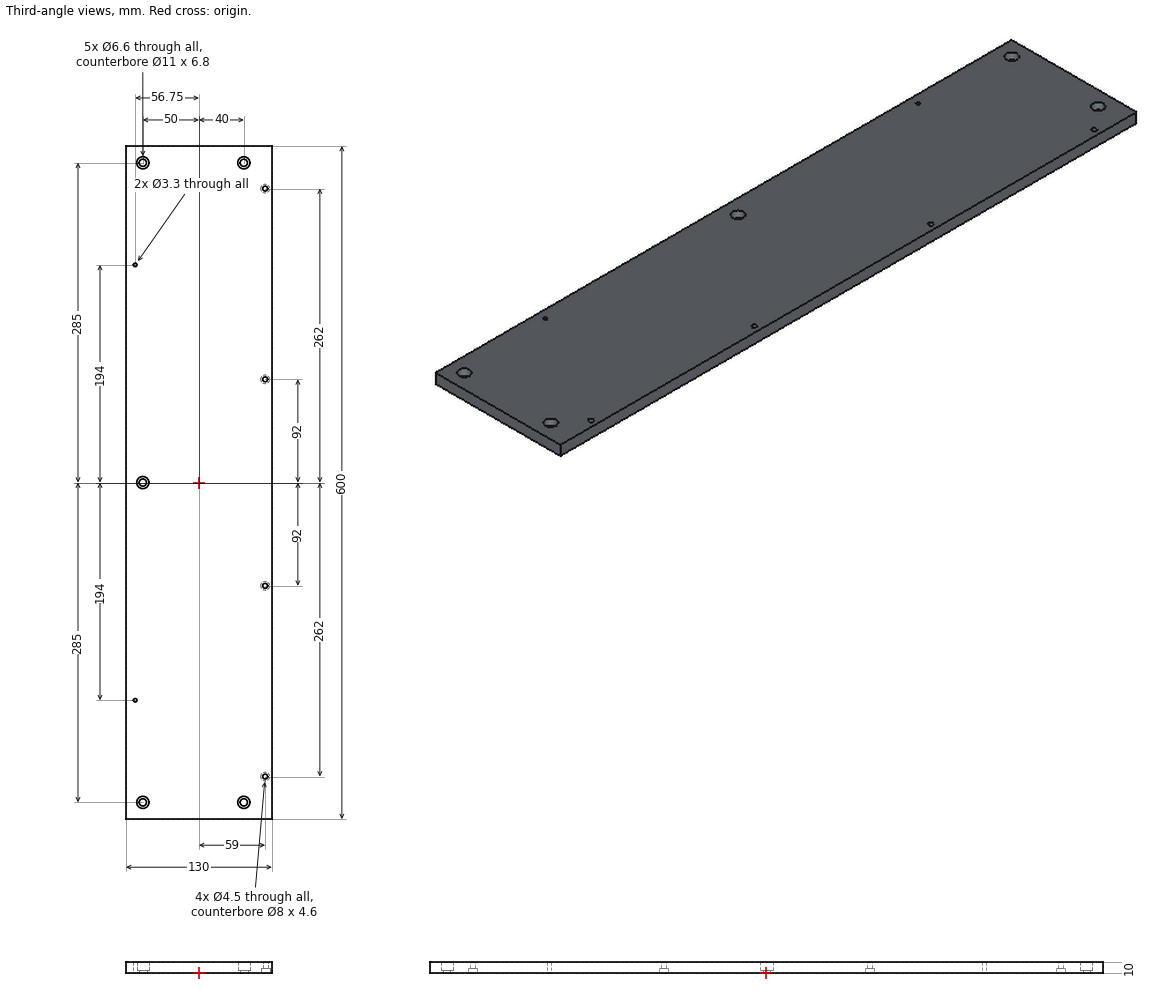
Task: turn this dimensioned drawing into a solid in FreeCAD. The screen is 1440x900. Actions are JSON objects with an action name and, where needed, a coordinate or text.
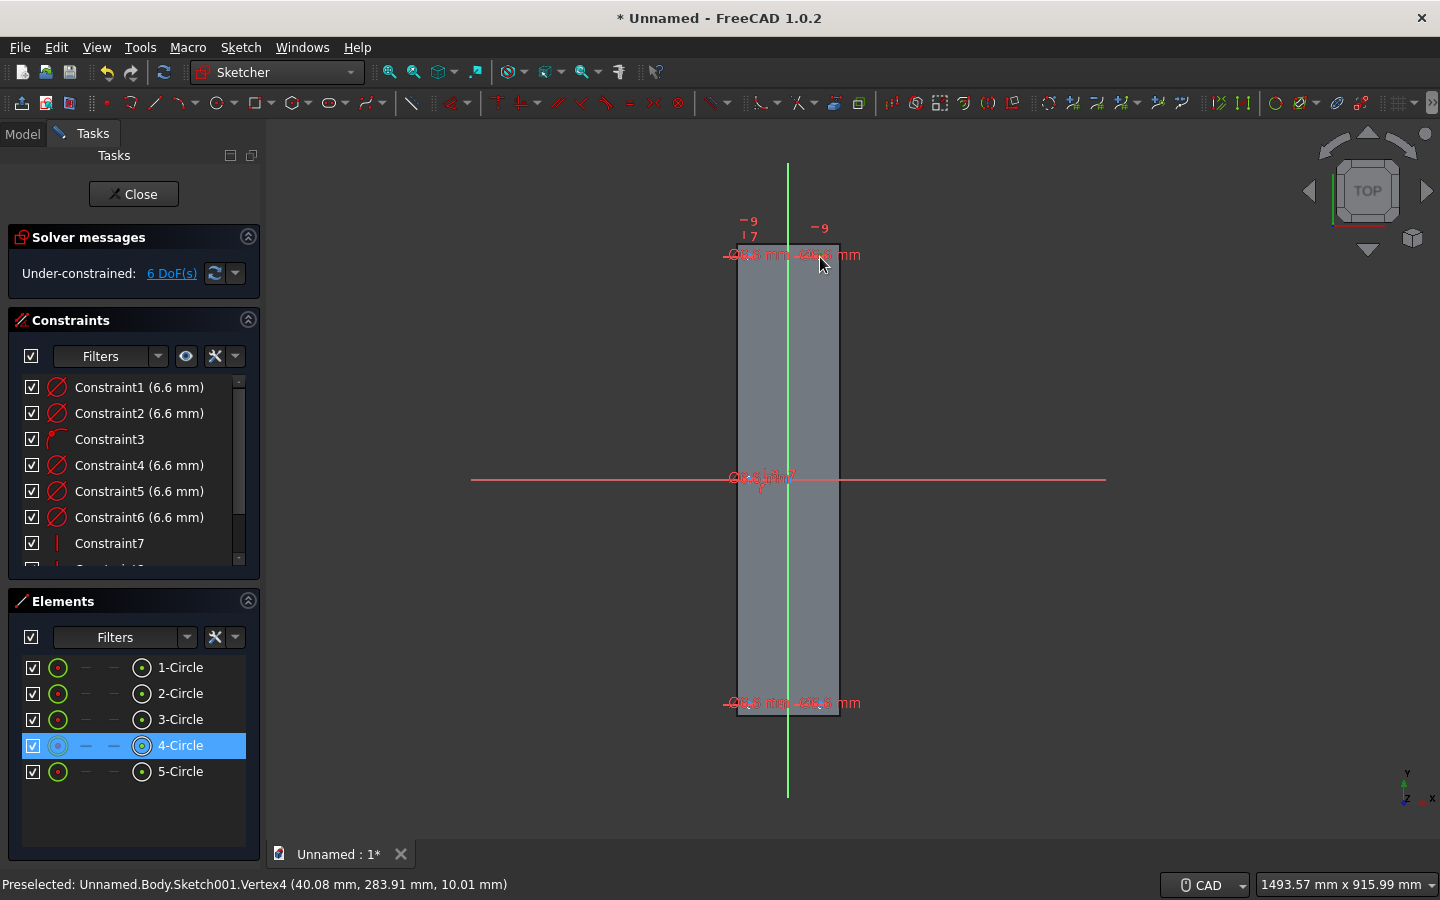
{"action": "left_click", "coordinate": [820, 705]}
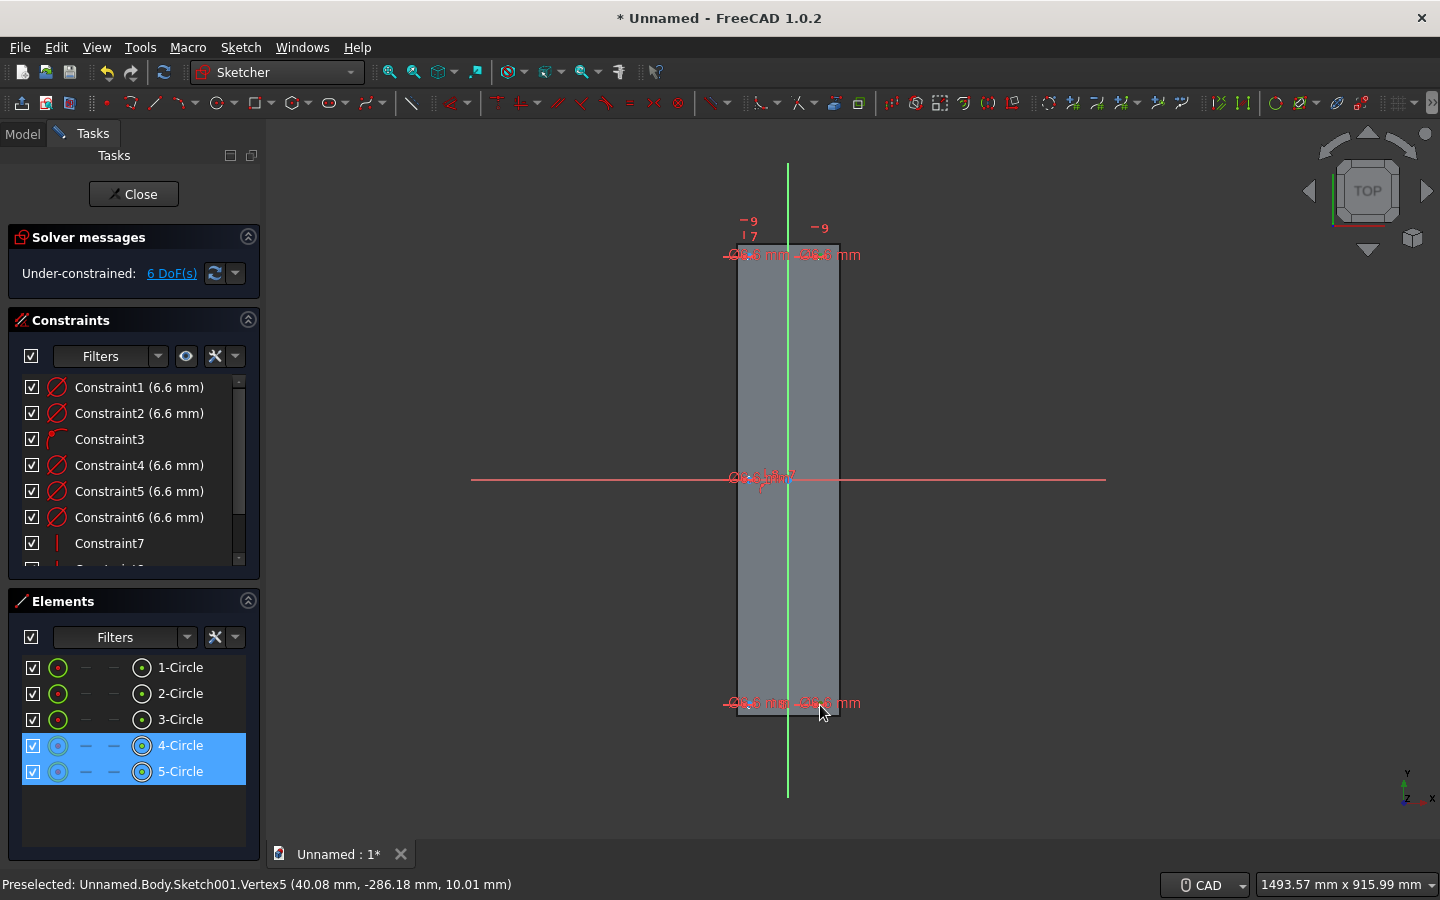
{"action": "key", "text": "v"}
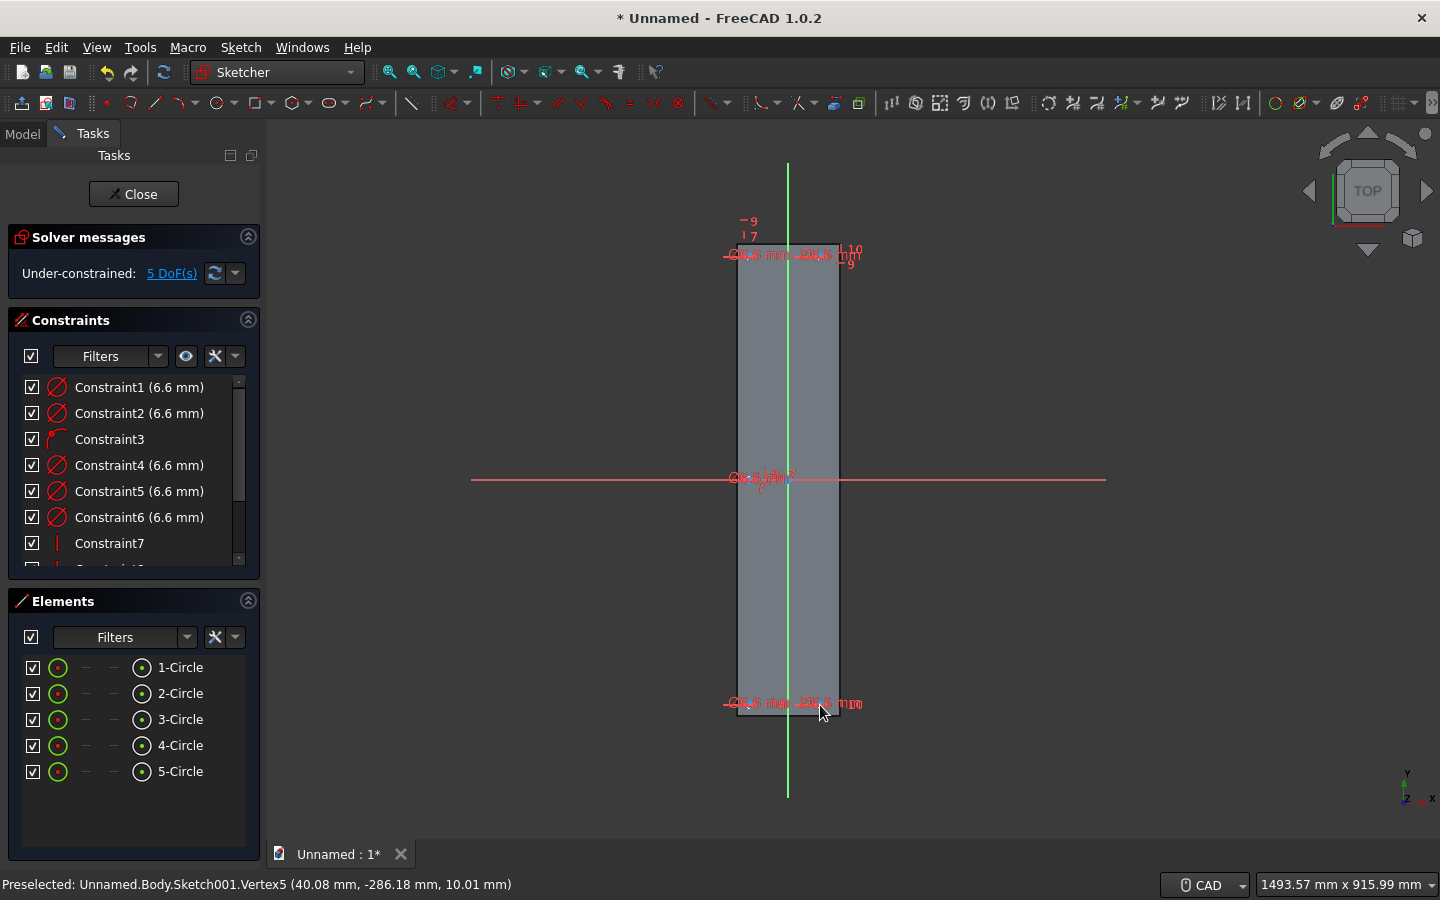
{"action": "left_click", "coordinate": [749, 705]}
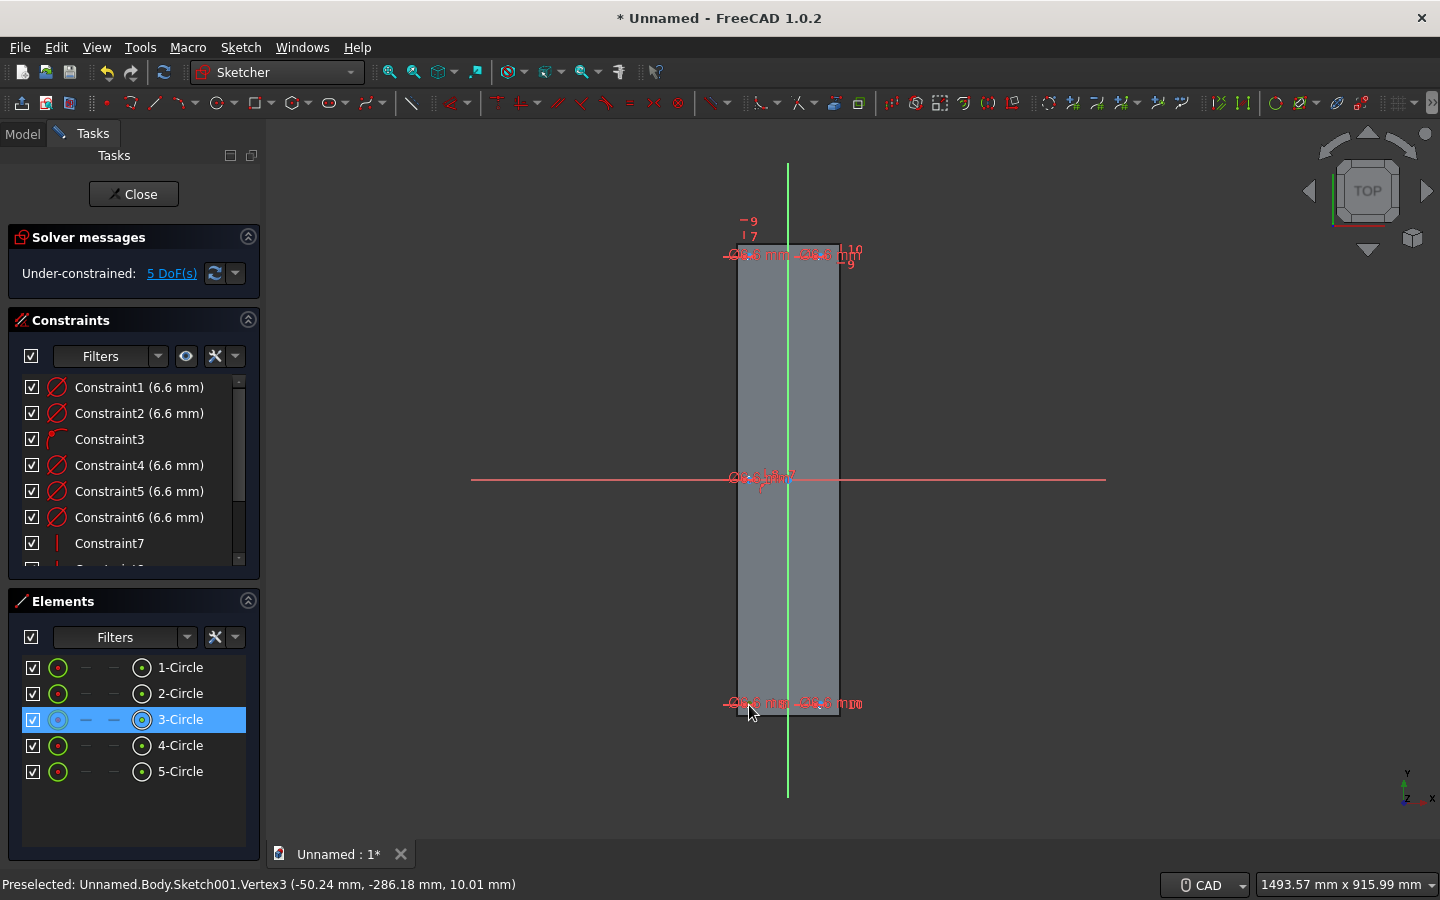
{"action": "left_click", "coordinate": [820, 705]}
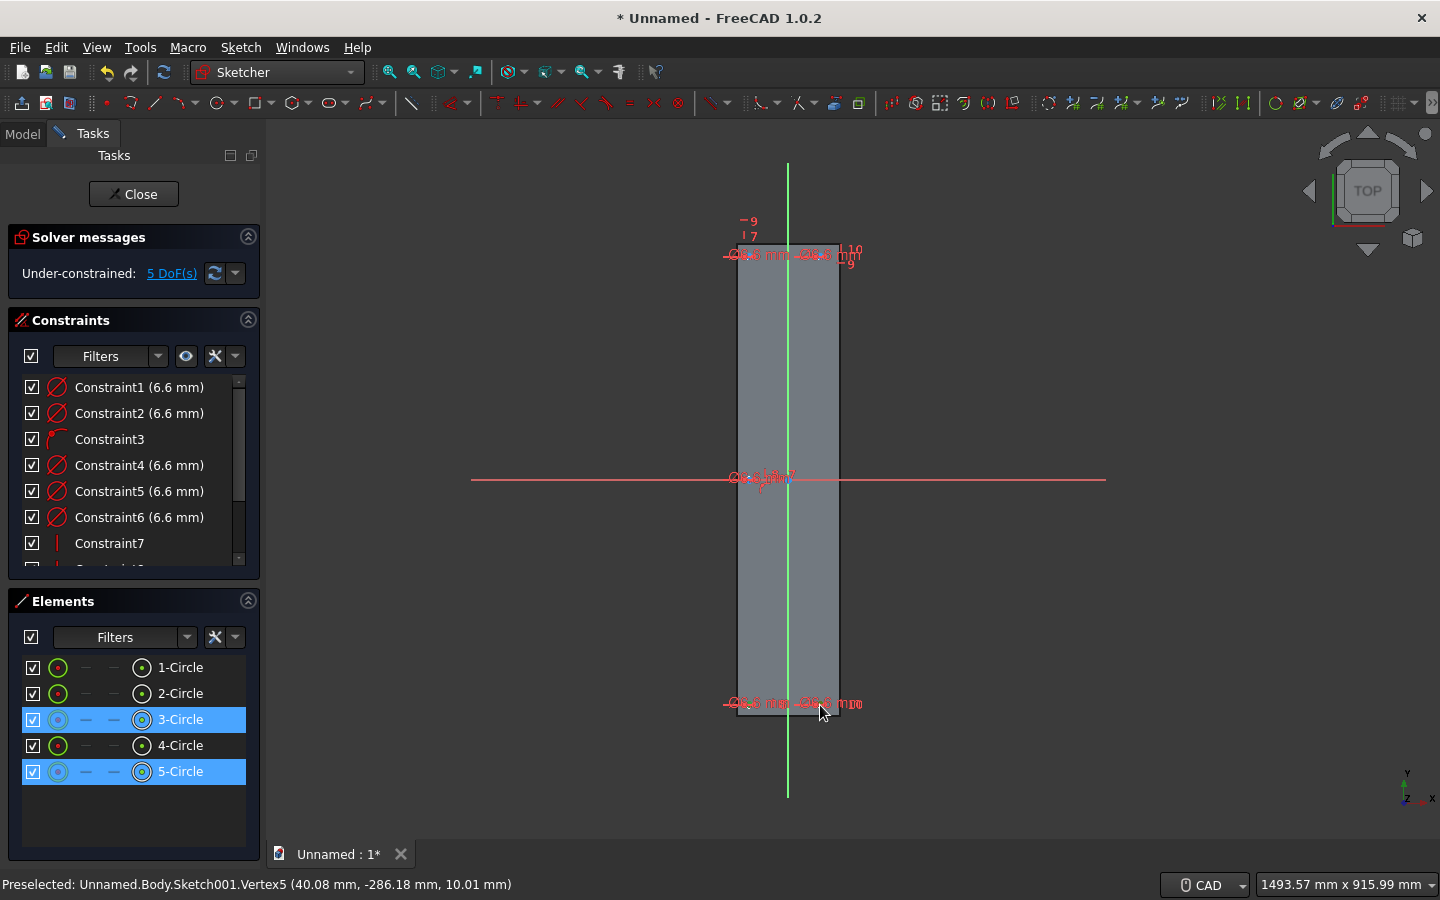
{"action": "left_click", "coordinate": [540, 104]}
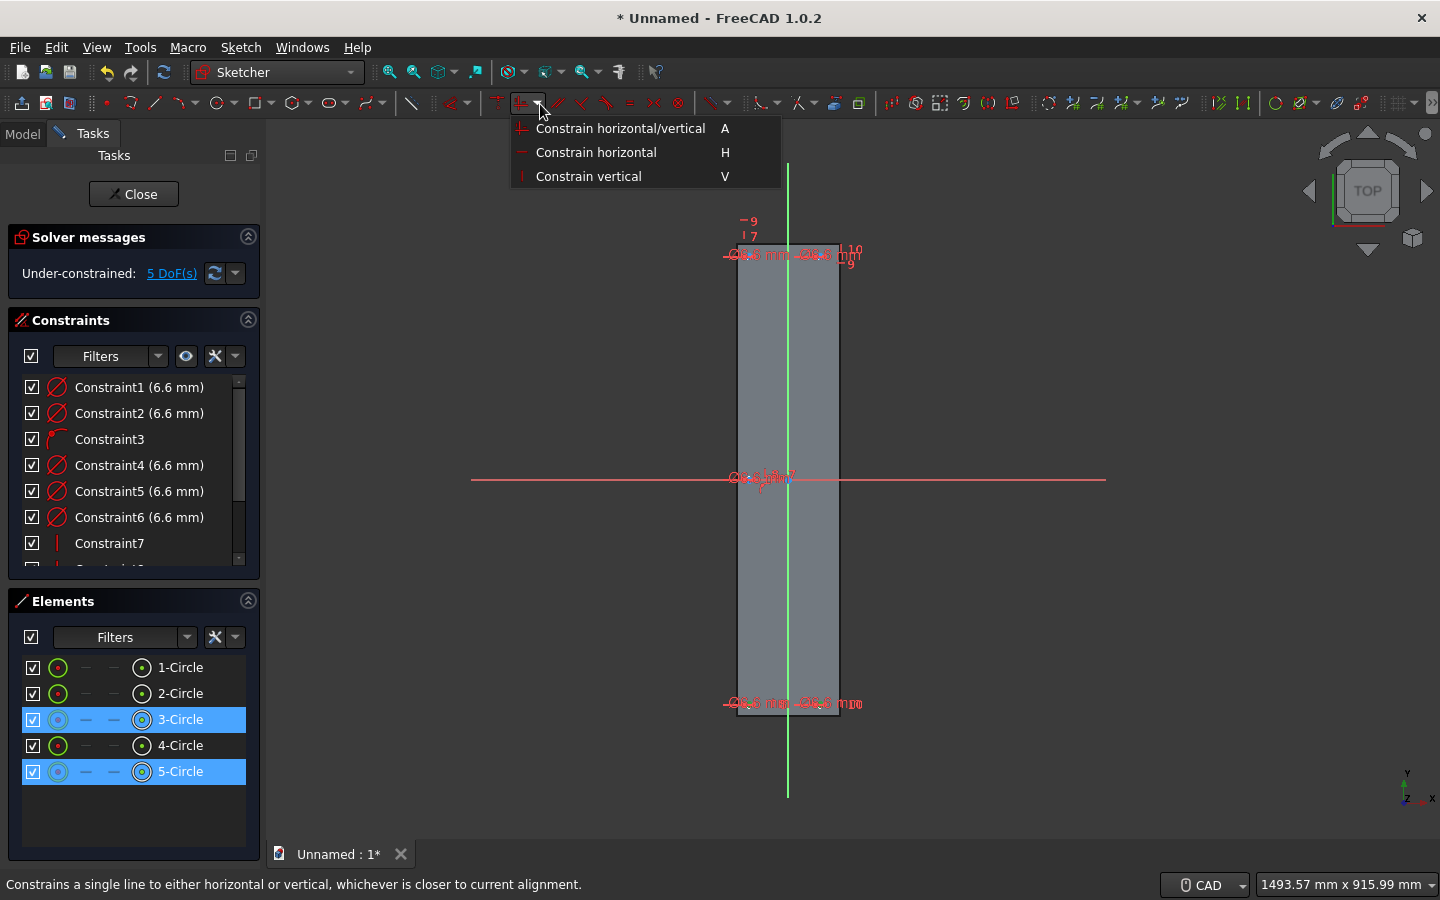
{"action": "left_click", "coordinate": [646, 152]}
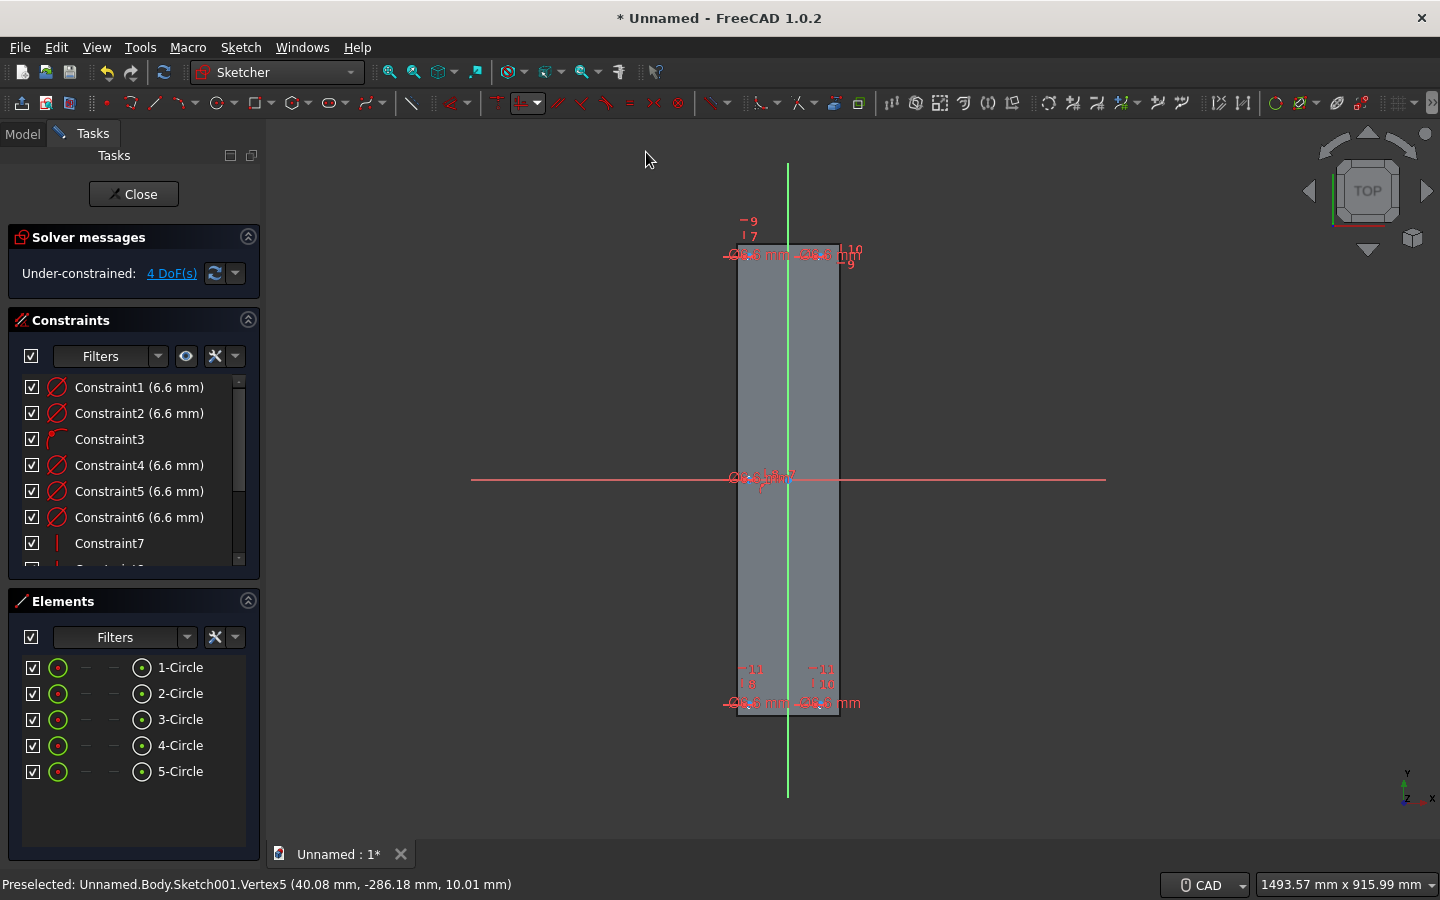
{"action": "key", "text": "d"}